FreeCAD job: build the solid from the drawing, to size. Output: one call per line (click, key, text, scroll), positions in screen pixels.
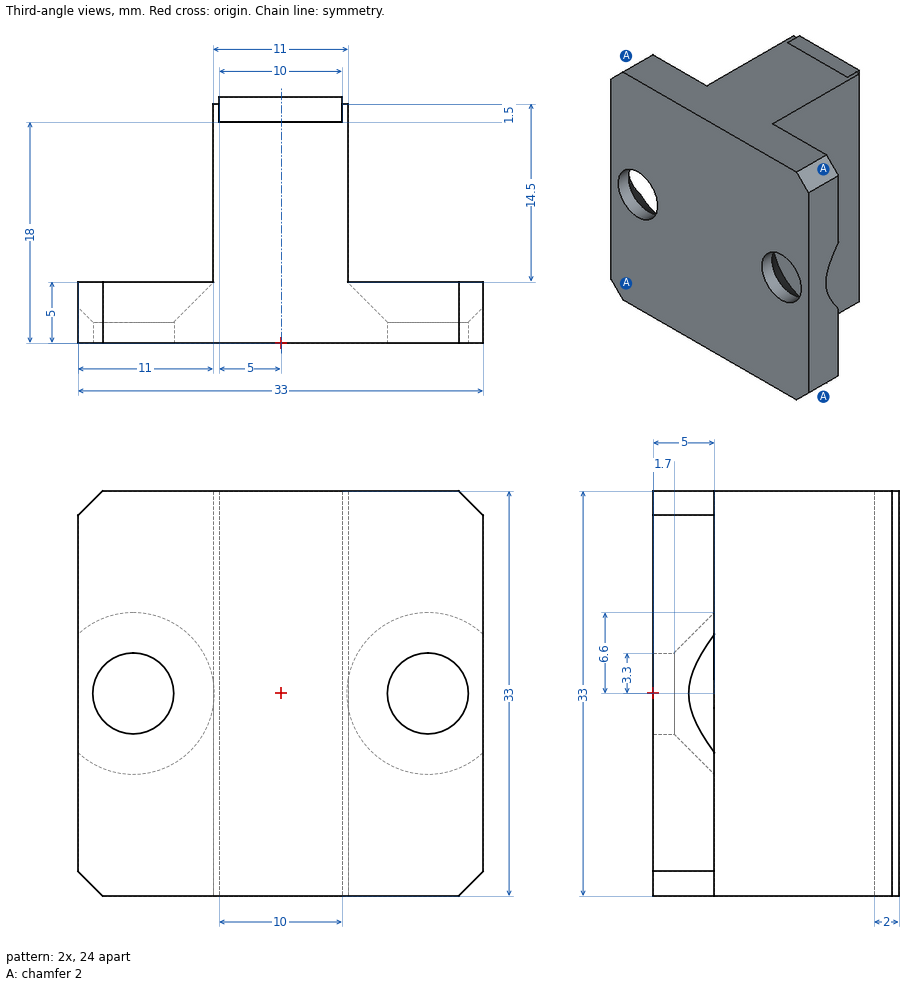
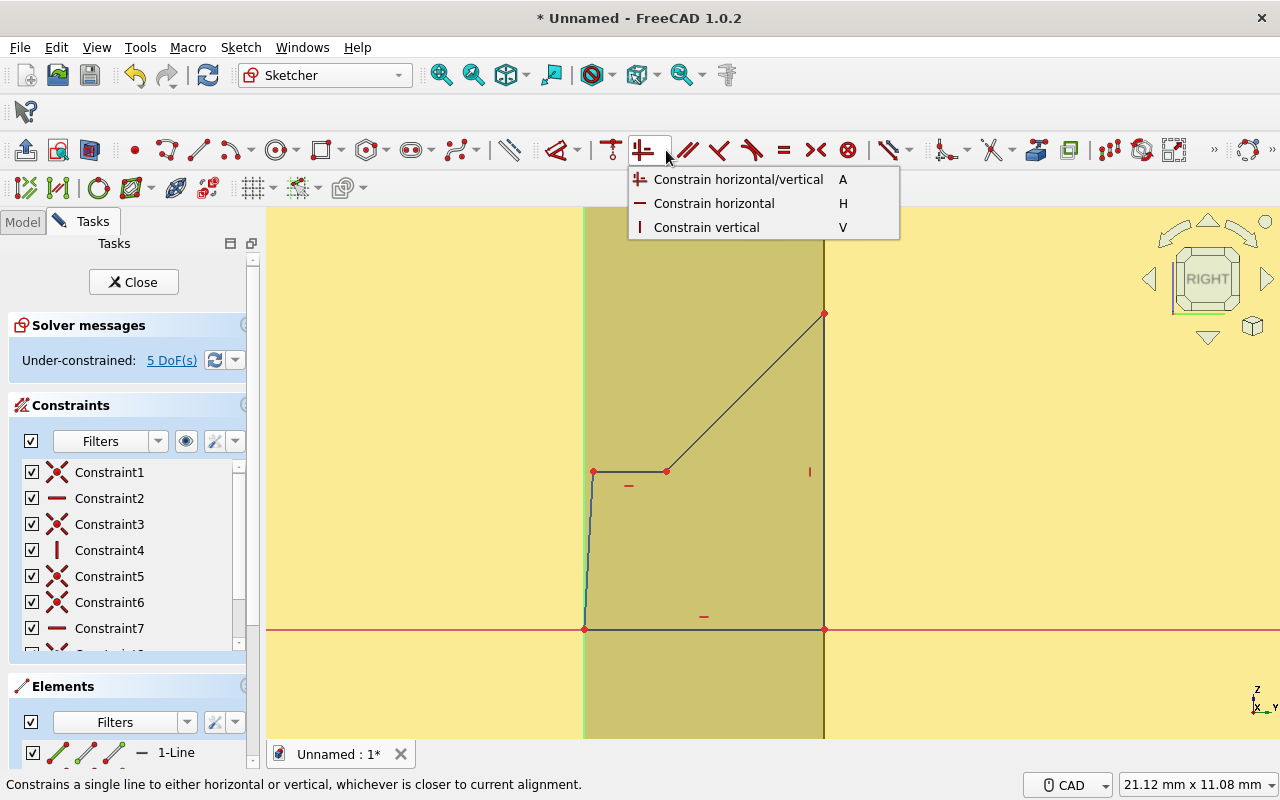
click(764, 227)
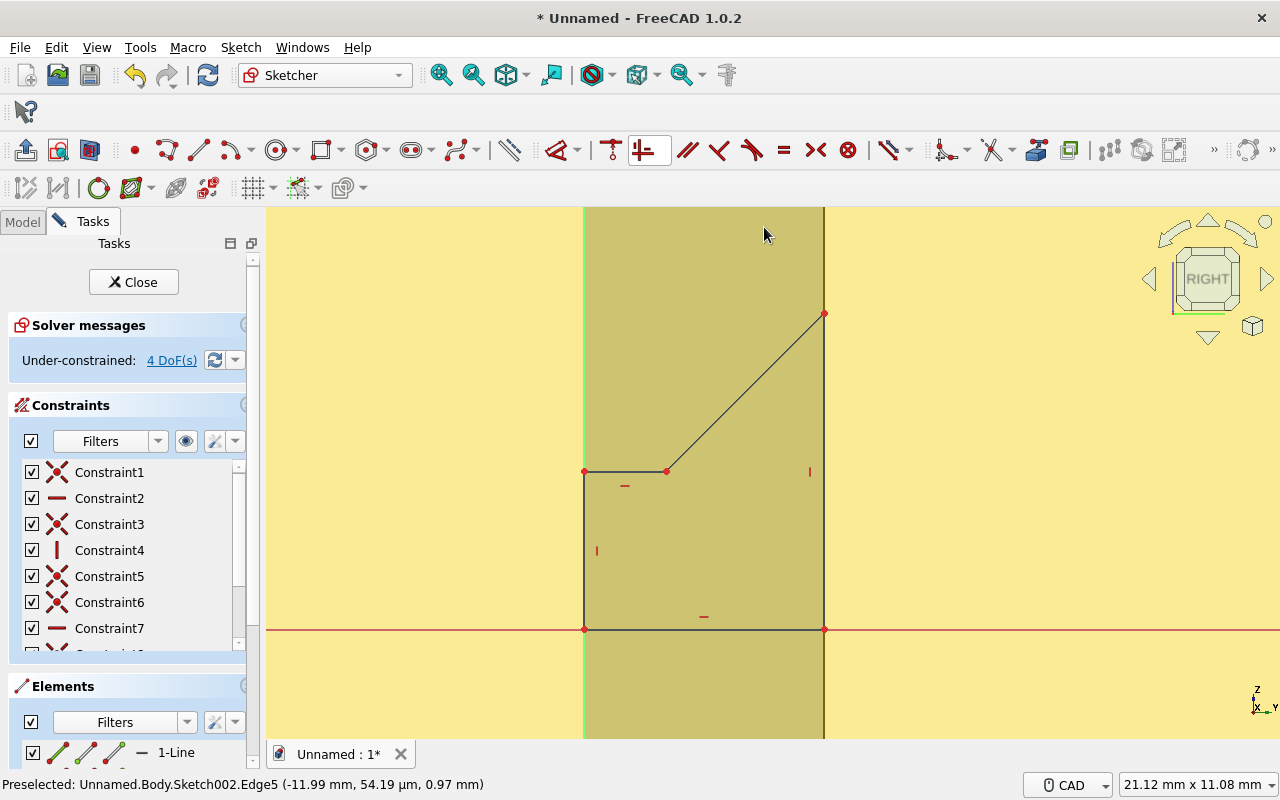
click(556, 150)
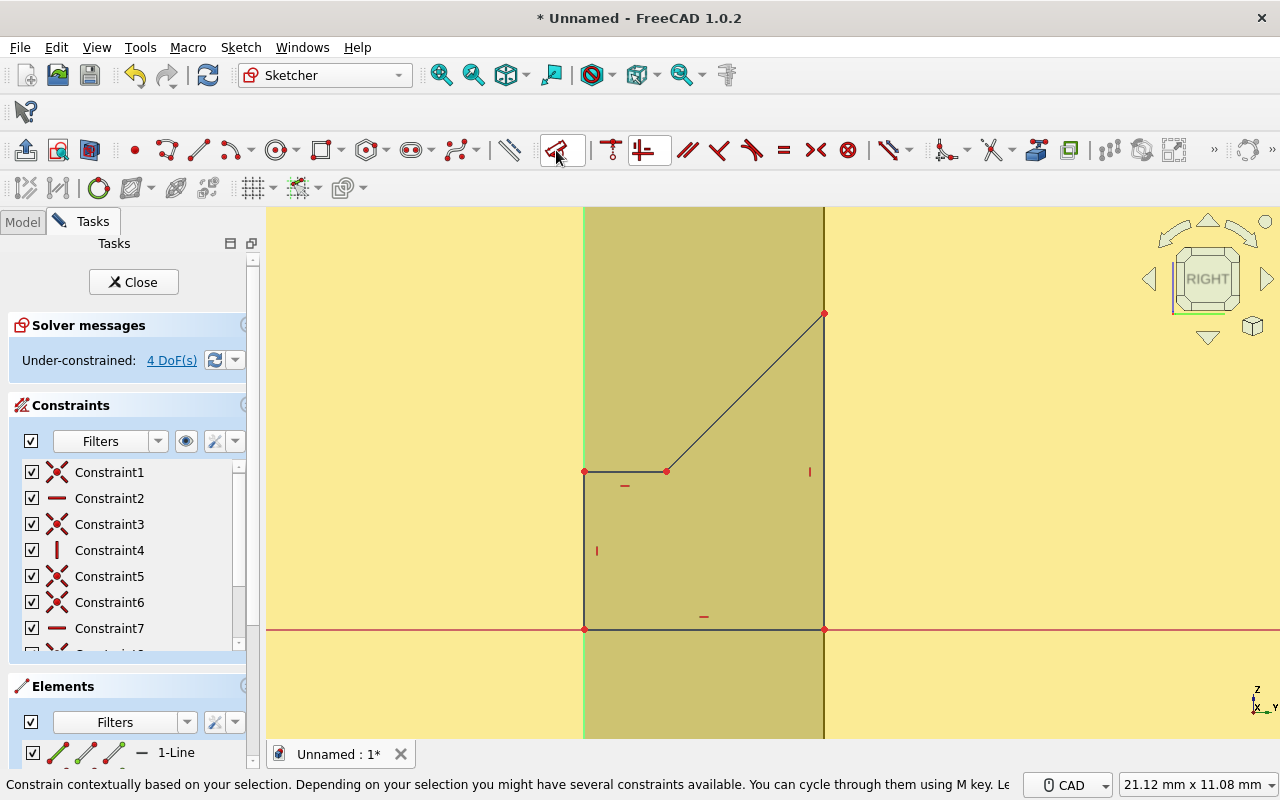
click(656, 630)
click(704, 664)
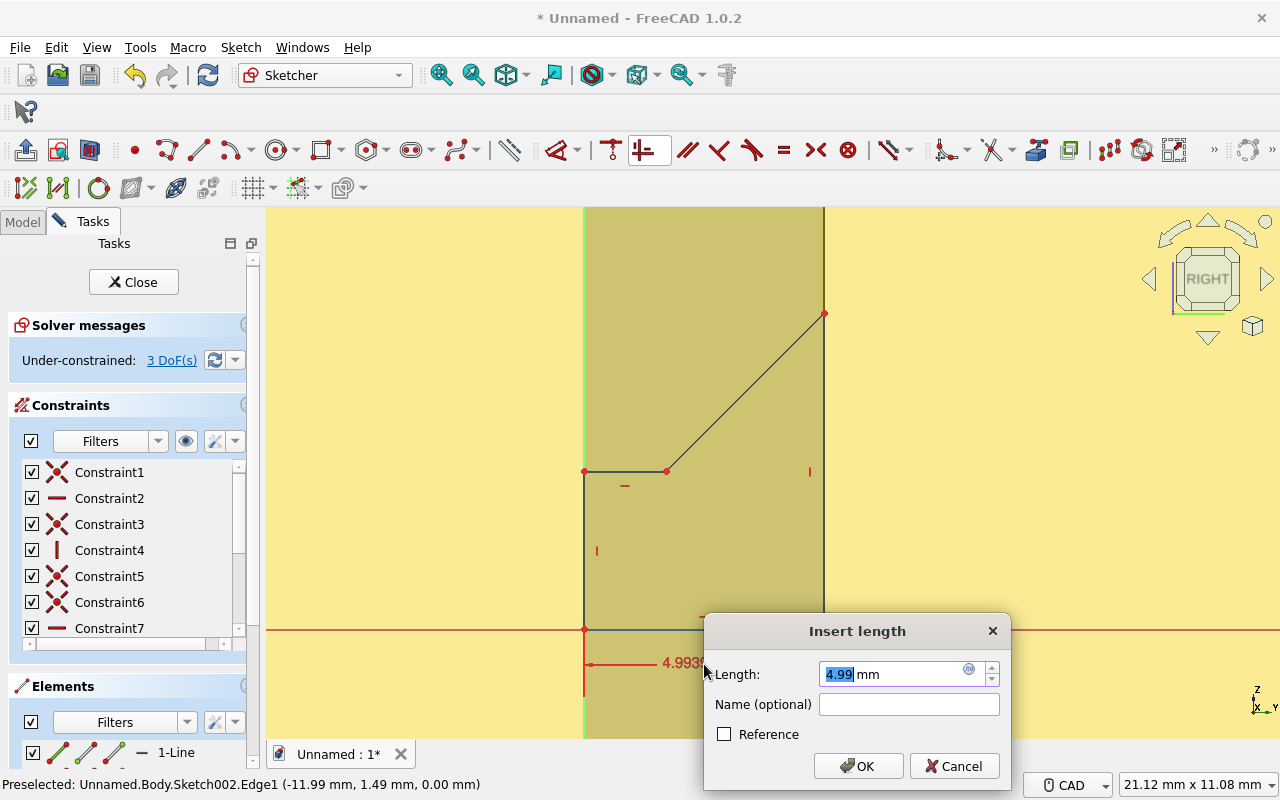
text(5)
key(Return)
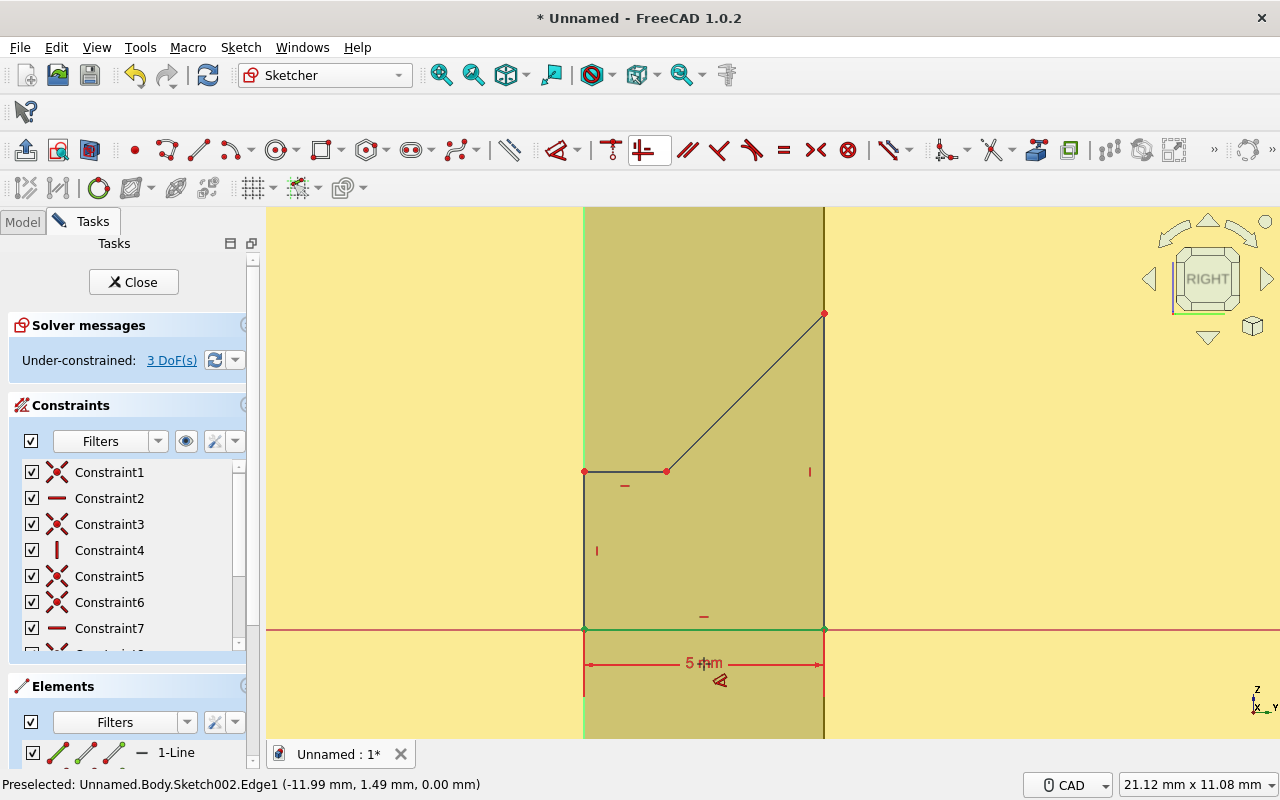
click(824, 535)
click(858, 472)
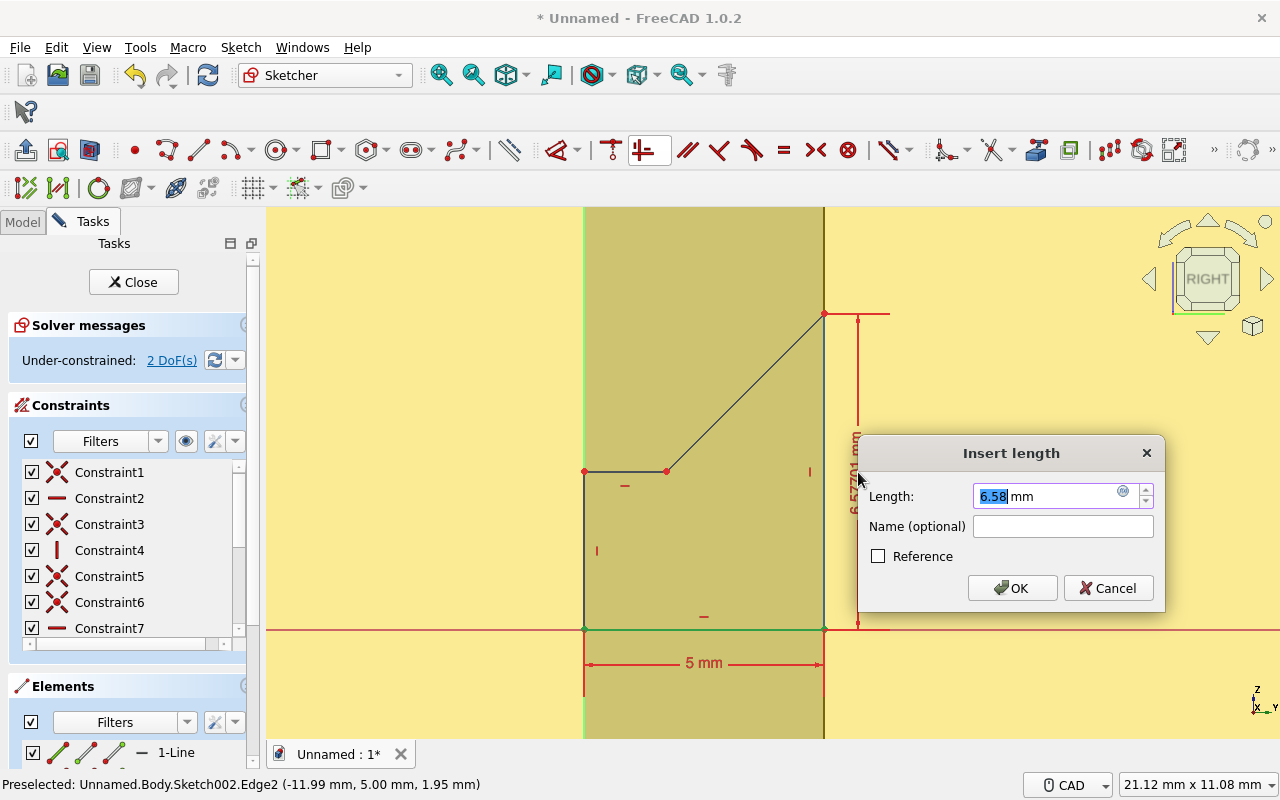
text(6.6)
key(Return)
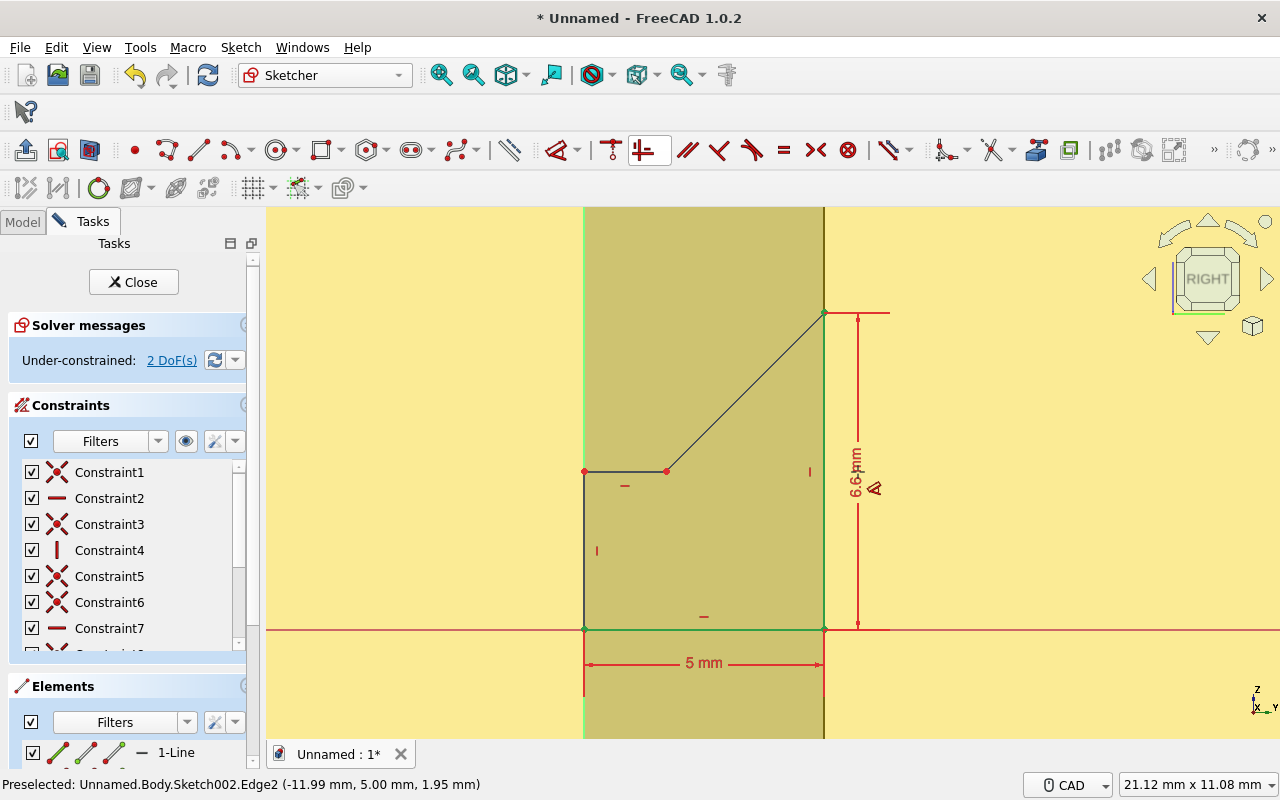
click(641, 472)
click(625, 506)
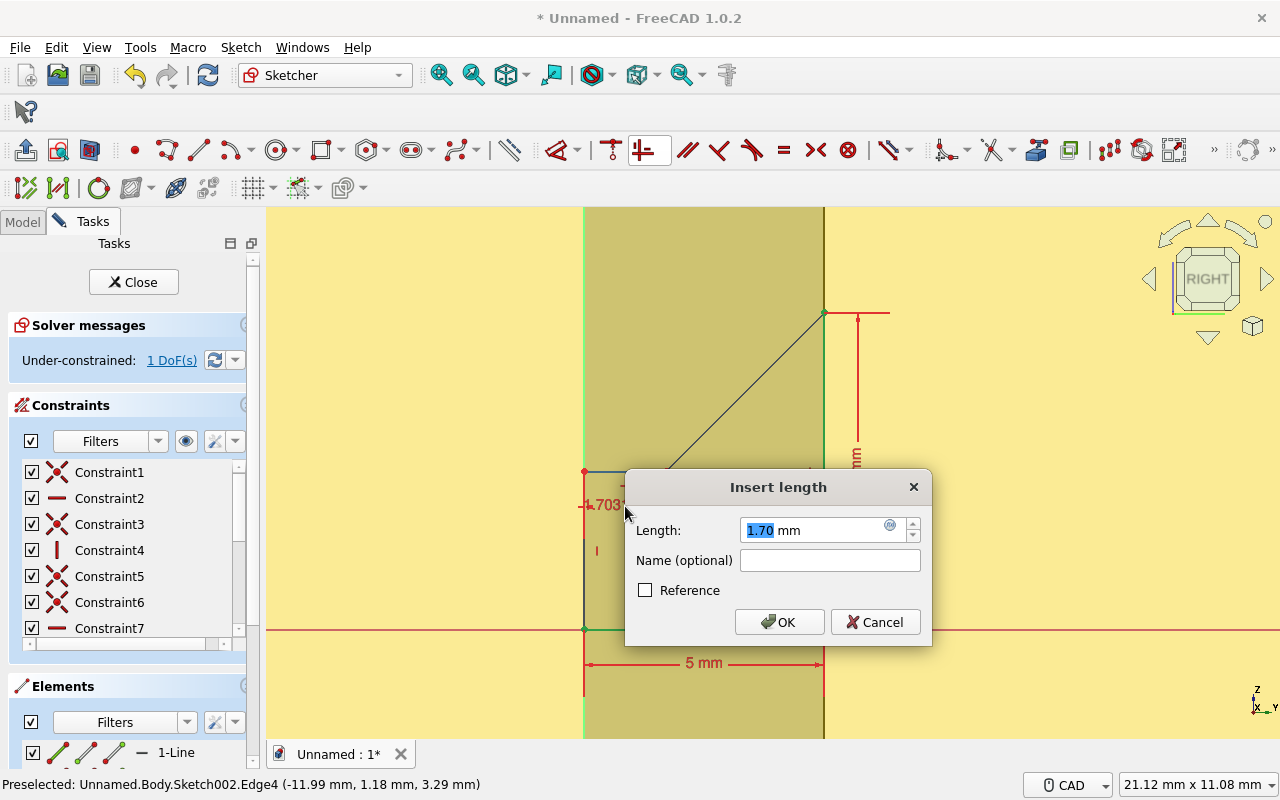
text(1.7)
key(Return)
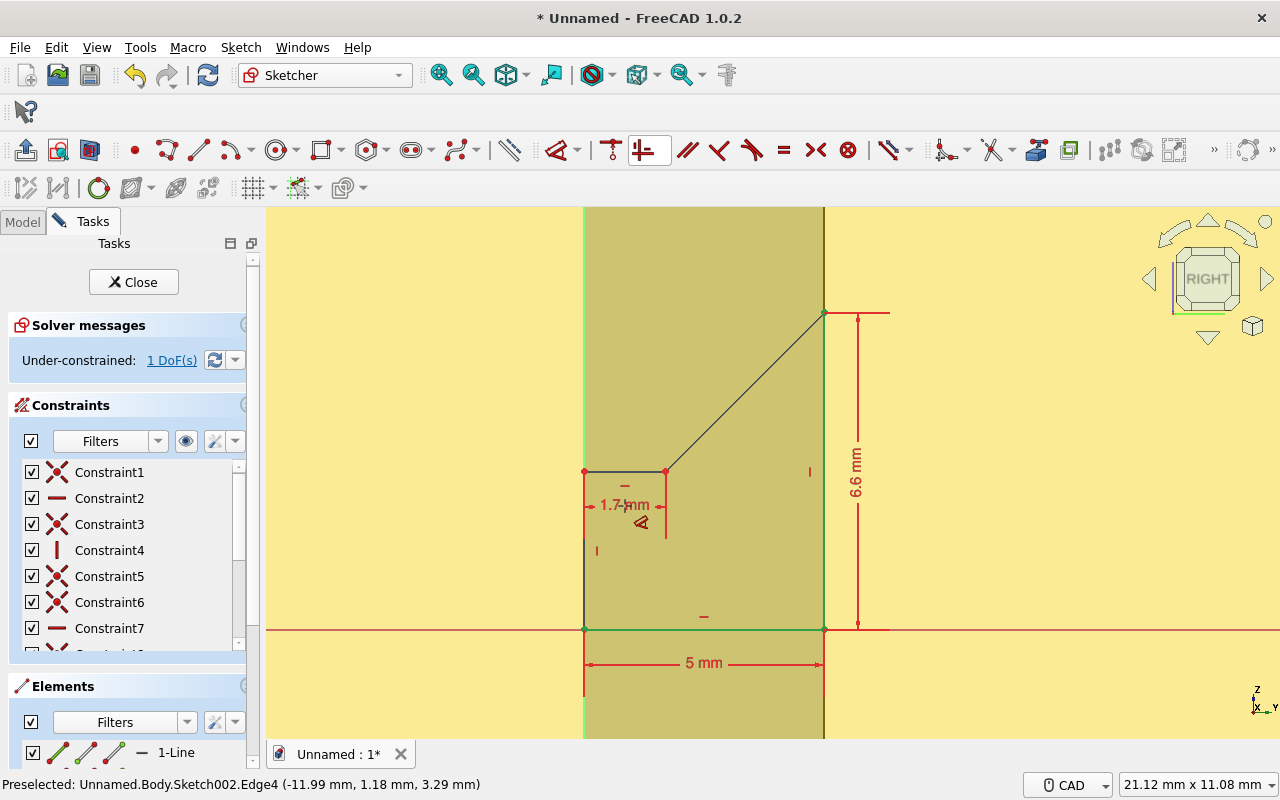
click(584, 519)
click(550, 551)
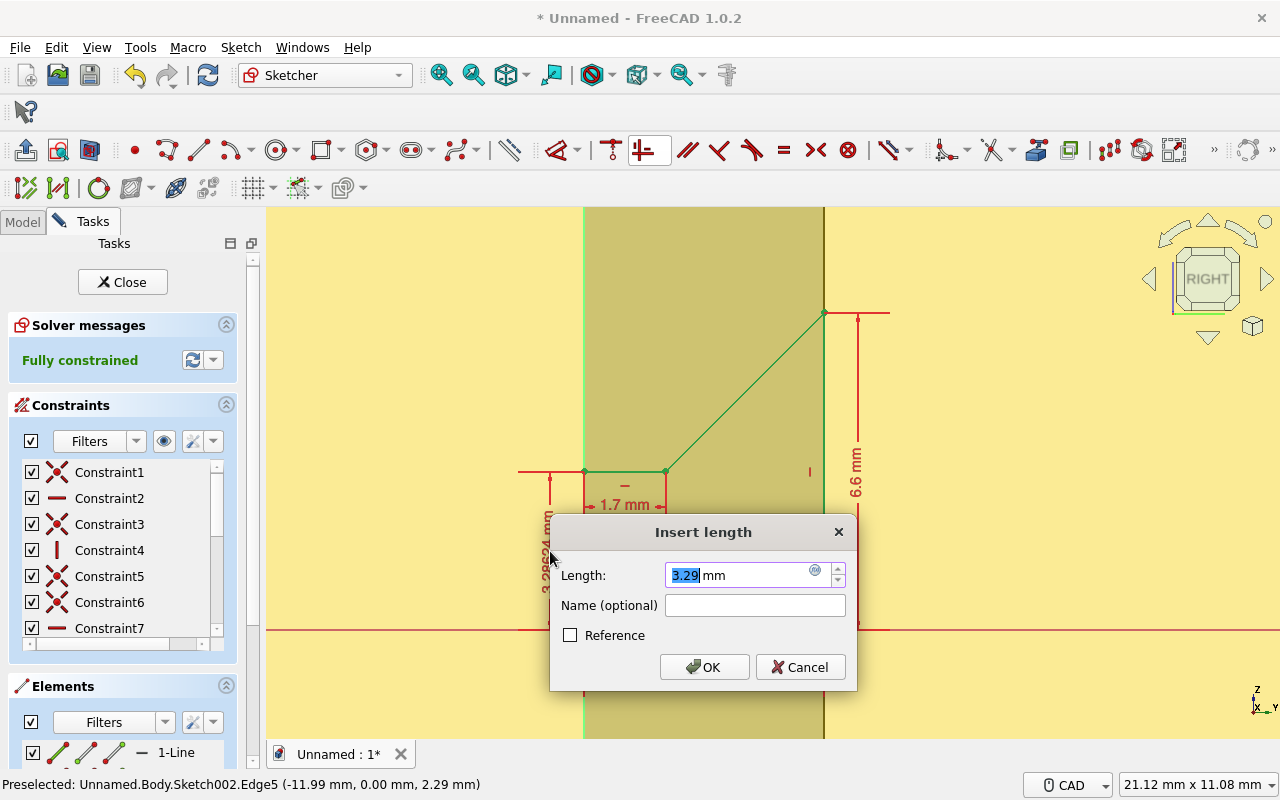
text(3.3)
key(Return)
key(Escape)